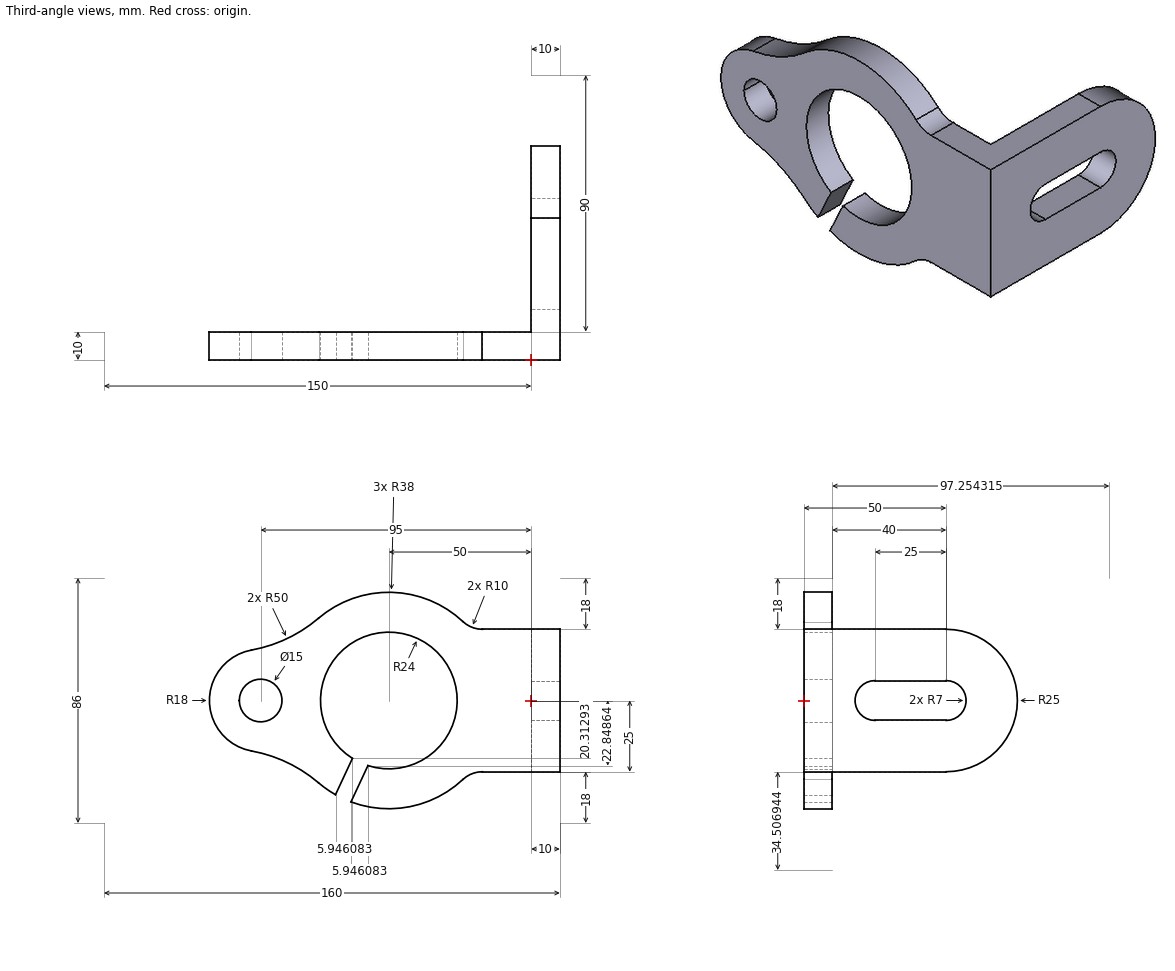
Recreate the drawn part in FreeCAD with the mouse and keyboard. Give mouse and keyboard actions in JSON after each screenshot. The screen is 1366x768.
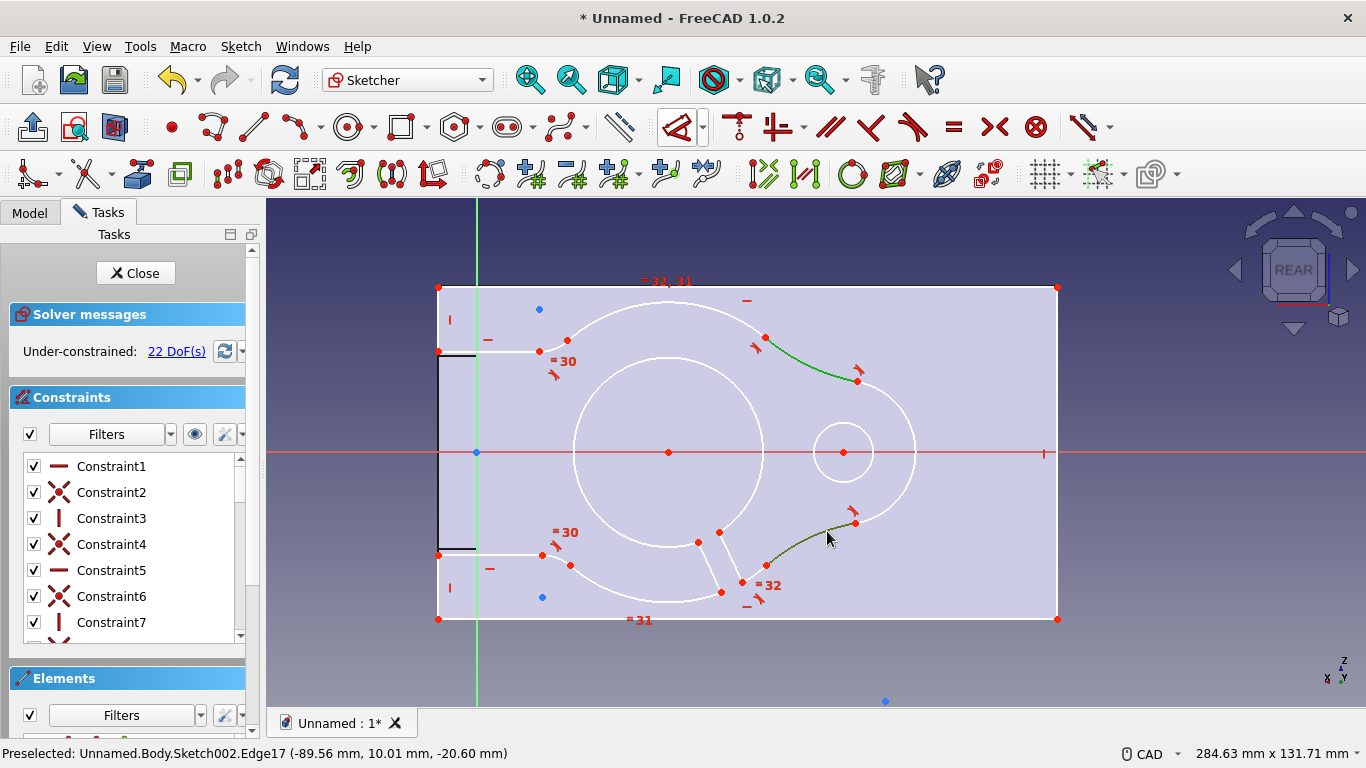
{"action": "key", "text": "e"}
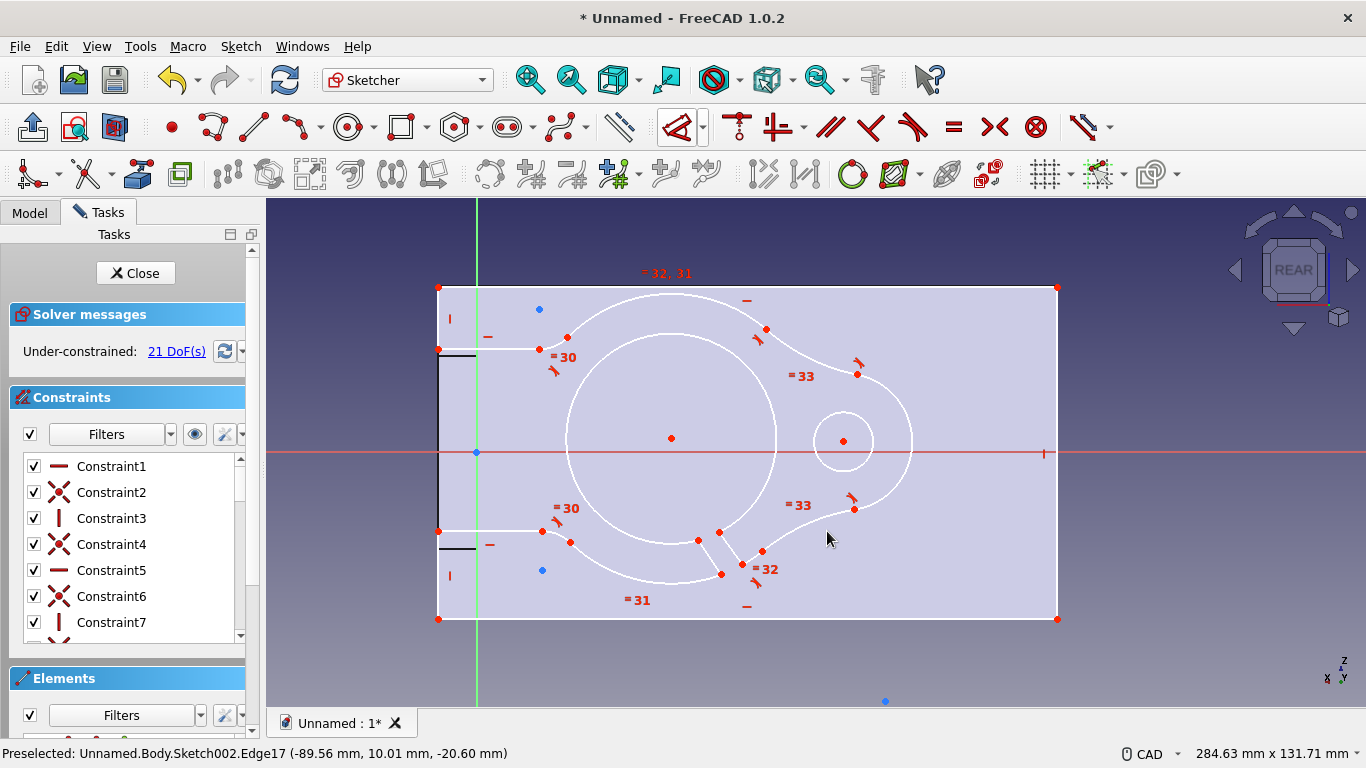
{"action": "left_click", "coordinate": [671, 439]}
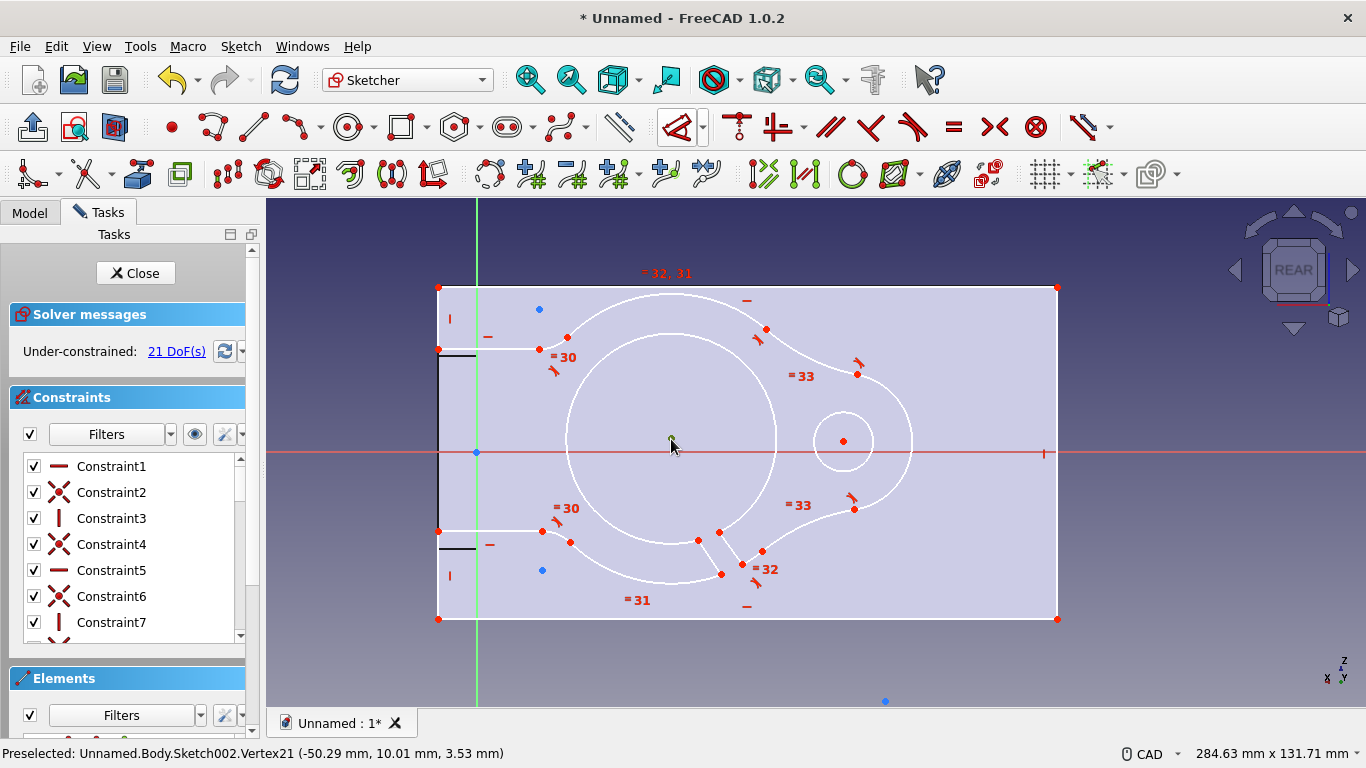
{"action": "left_click", "coordinate": [359, 452]}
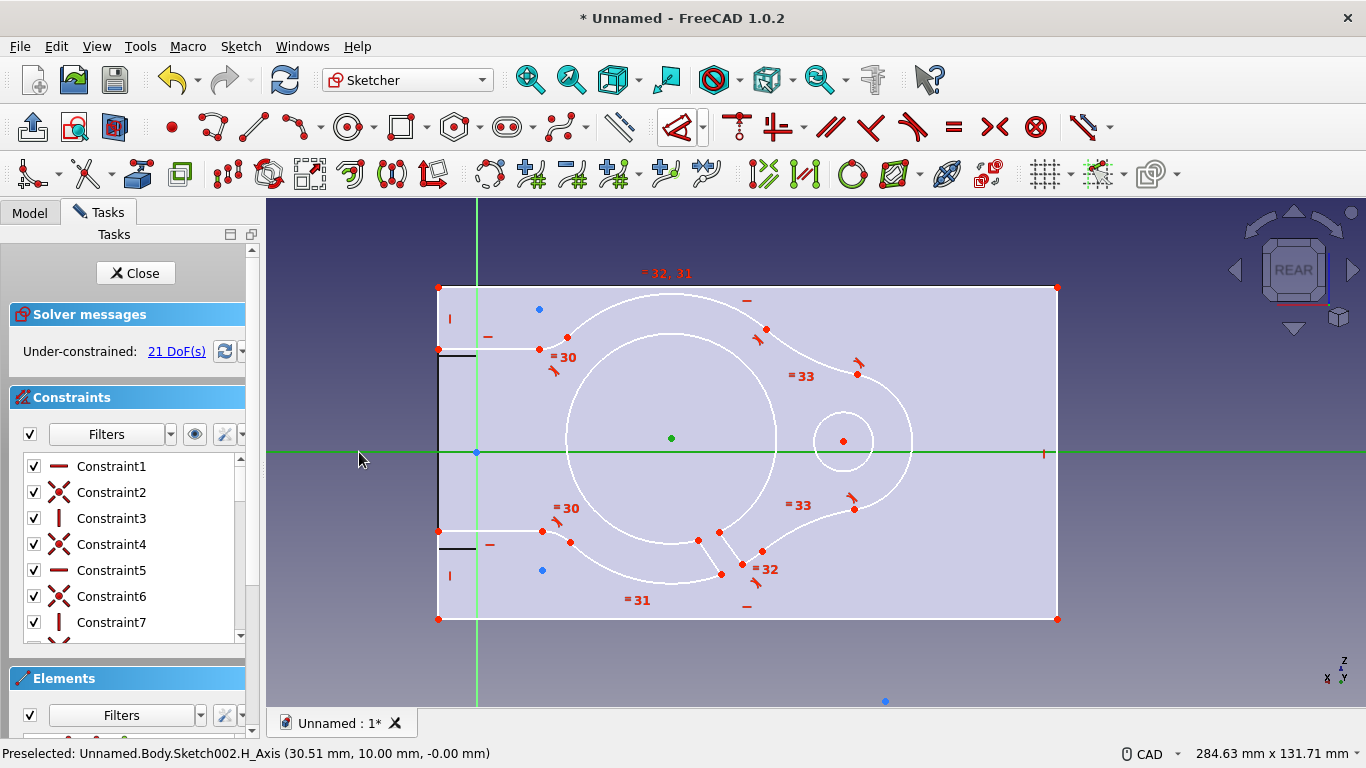
{"action": "left_click", "coordinate": [737, 128]}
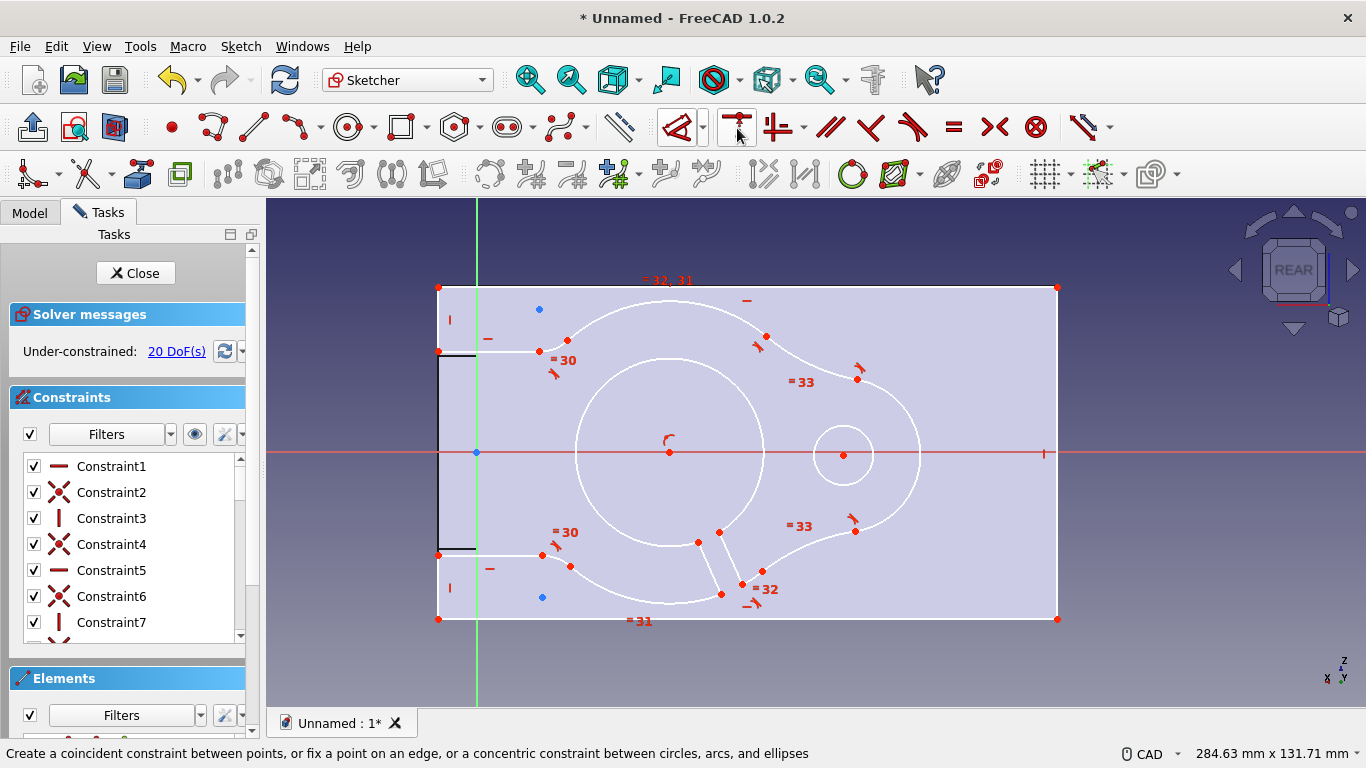
{"action": "left_click", "coordinate": [844, 455]}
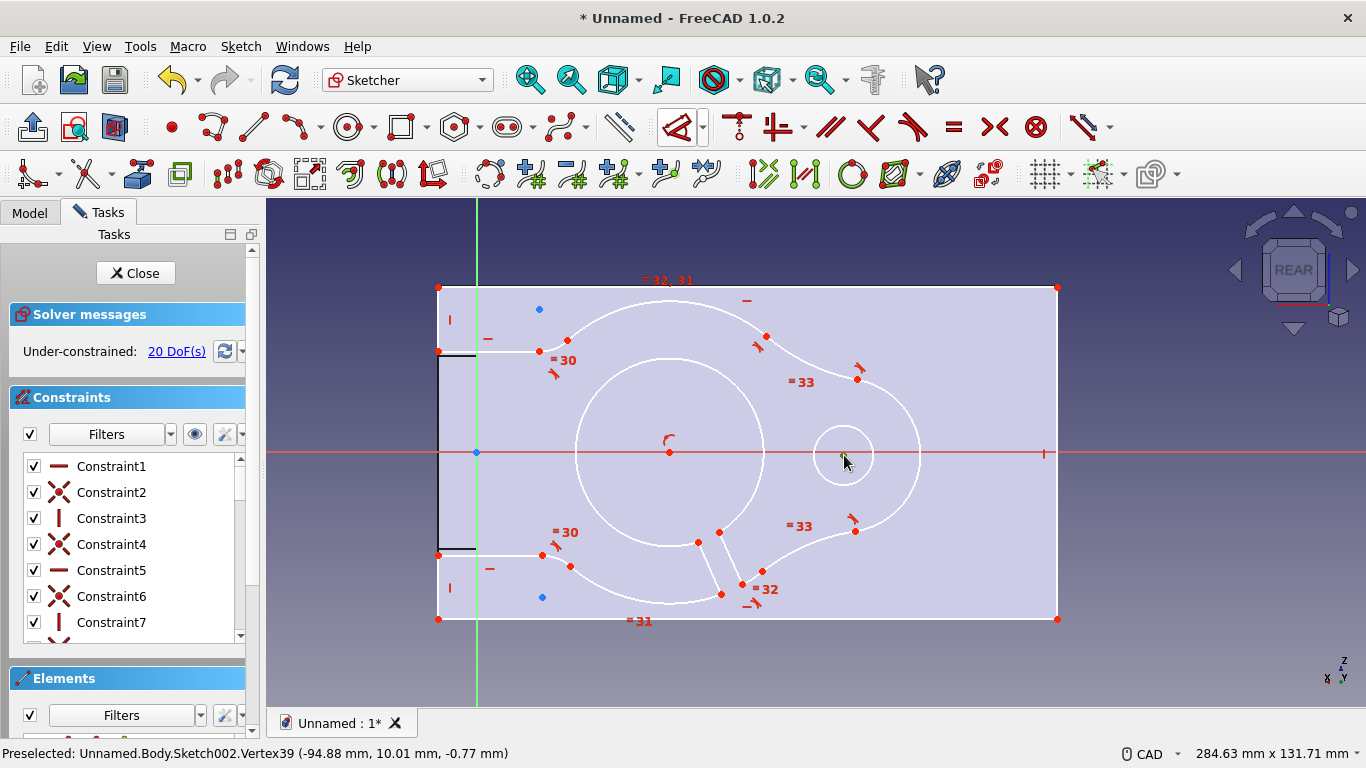
{"action": "left_click", "coordinate": [359, 452]}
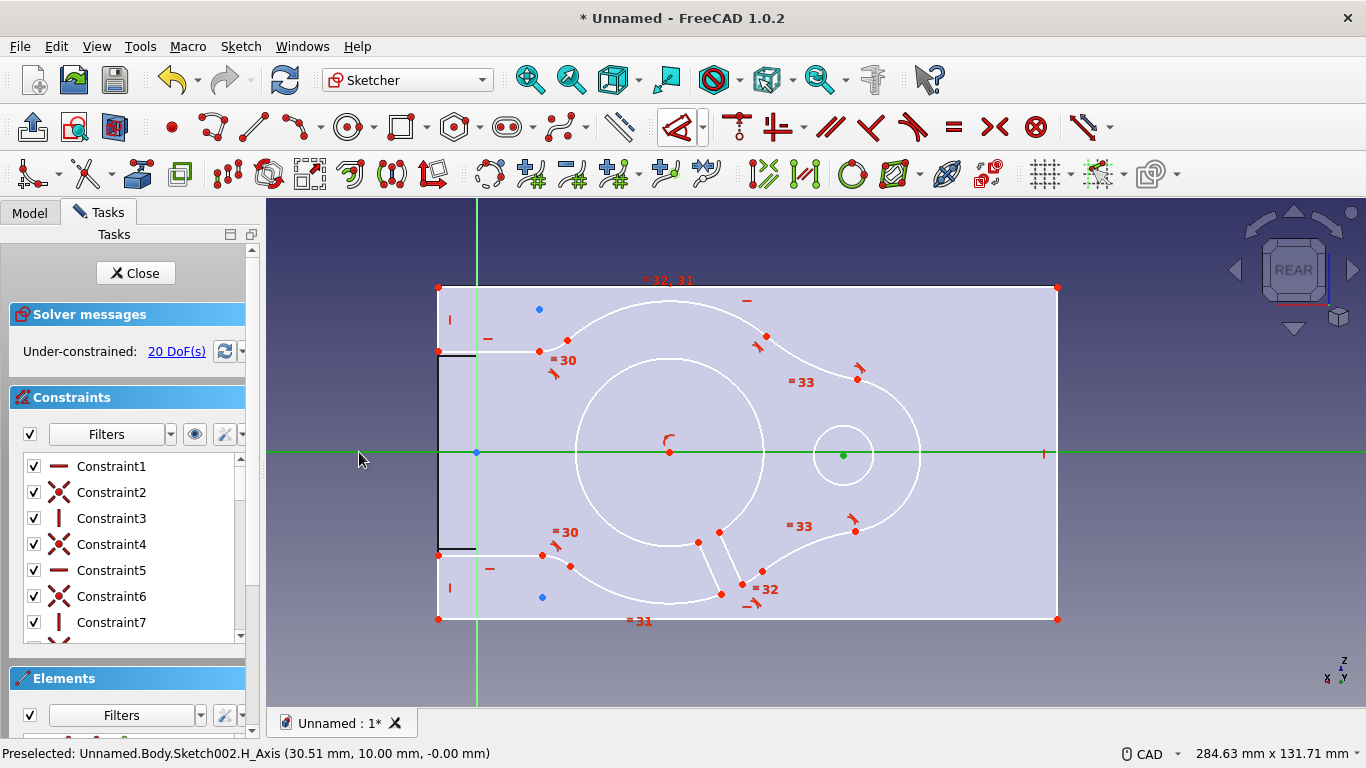
{"action": "left_click", "coordinate": [737, 128]}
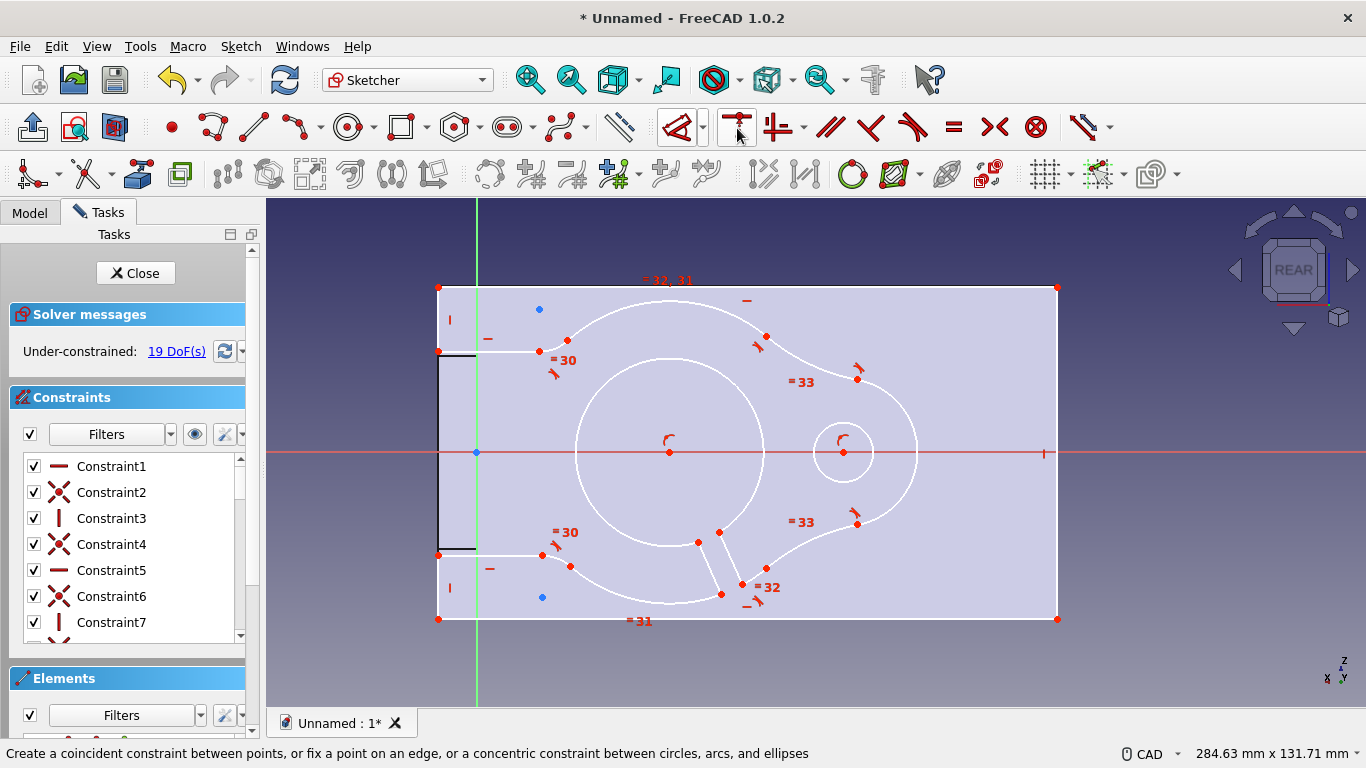
{"action": "left_click", "coordinate": [736, 385]}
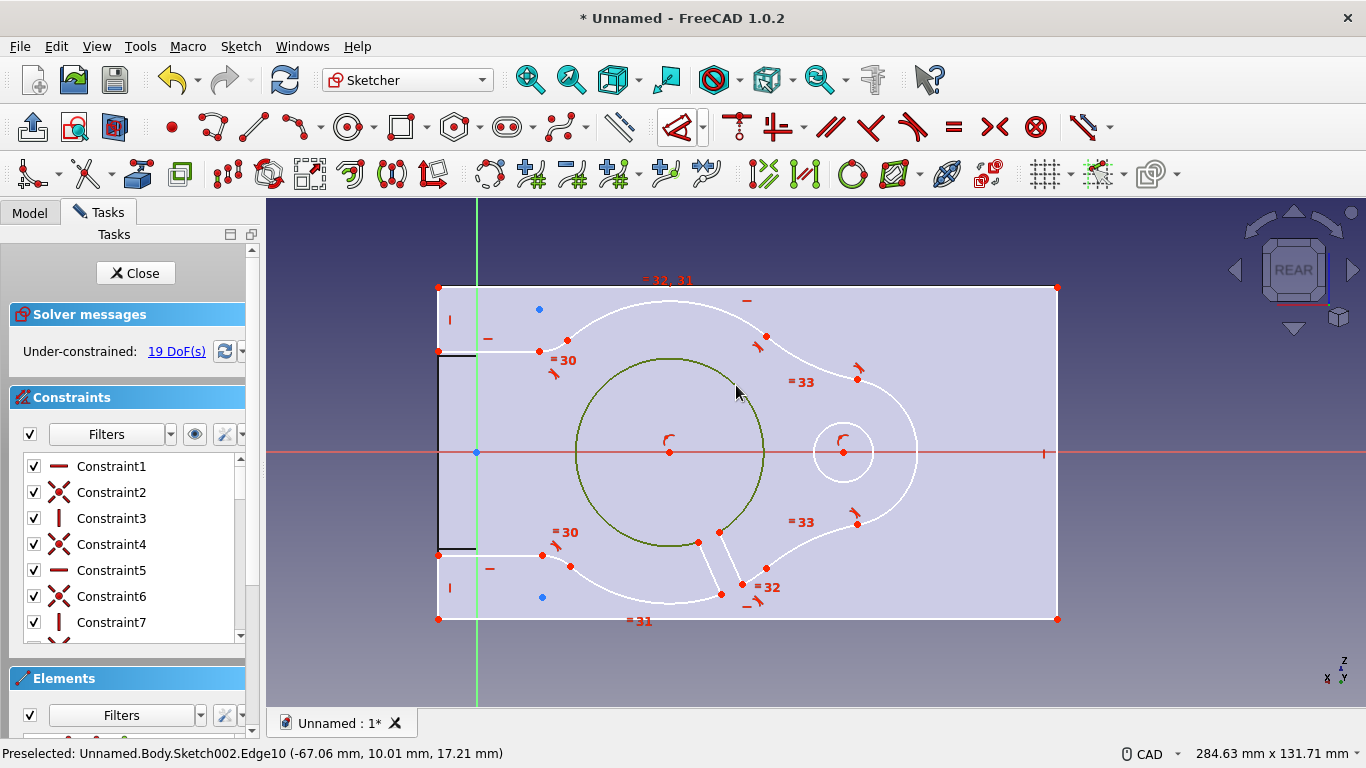
{"action": "left_click", "coordinate": [702, 128]}